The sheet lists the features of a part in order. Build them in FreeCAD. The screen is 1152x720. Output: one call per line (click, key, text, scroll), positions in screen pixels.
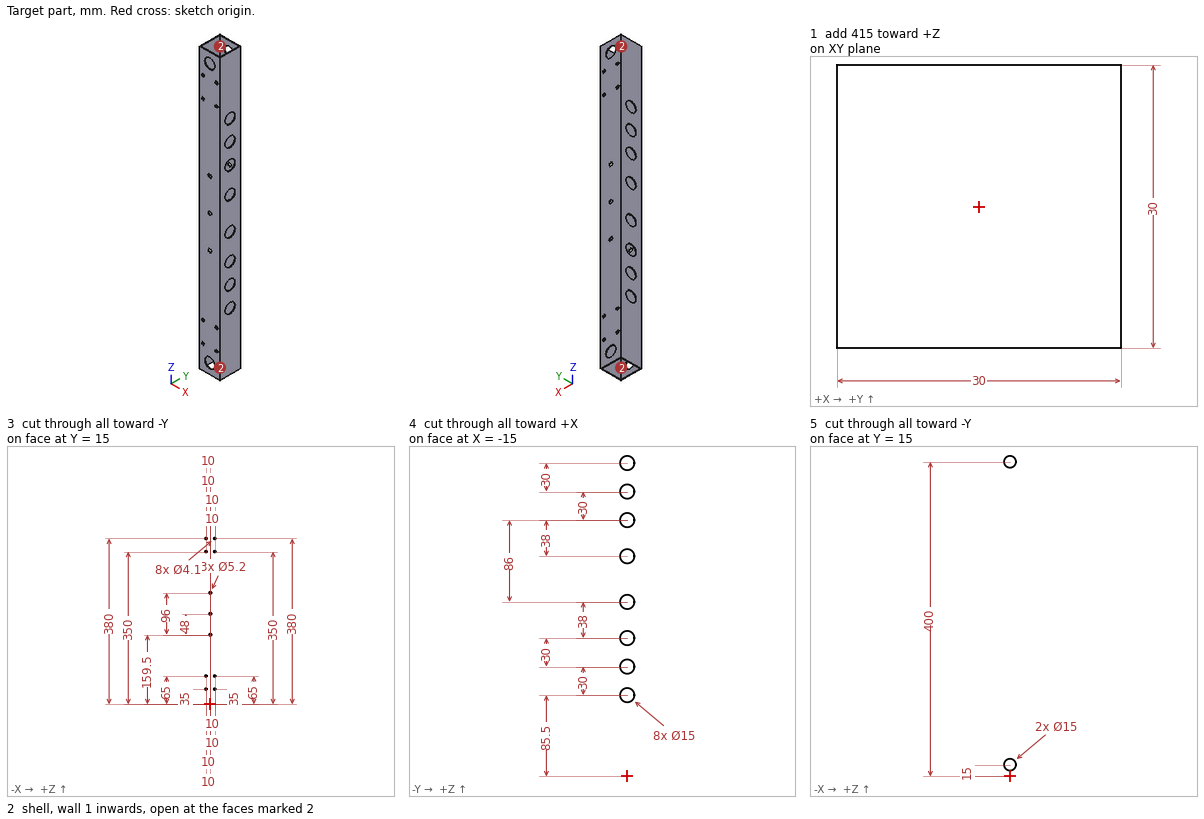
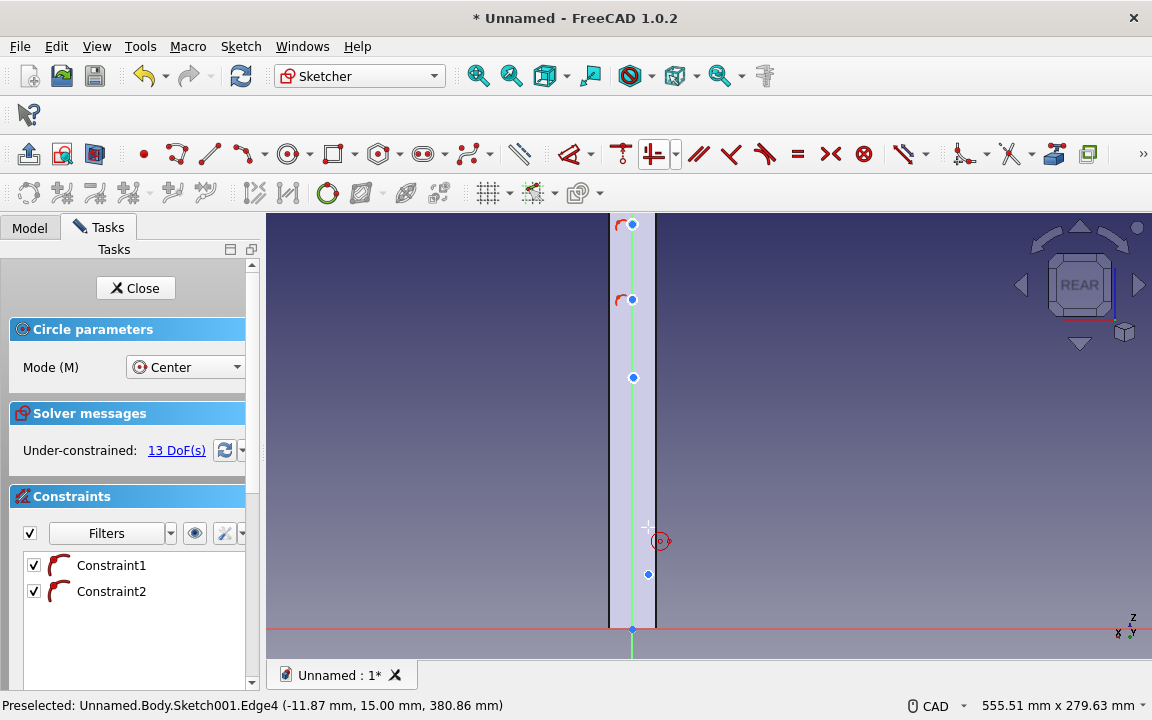
click(648, 526)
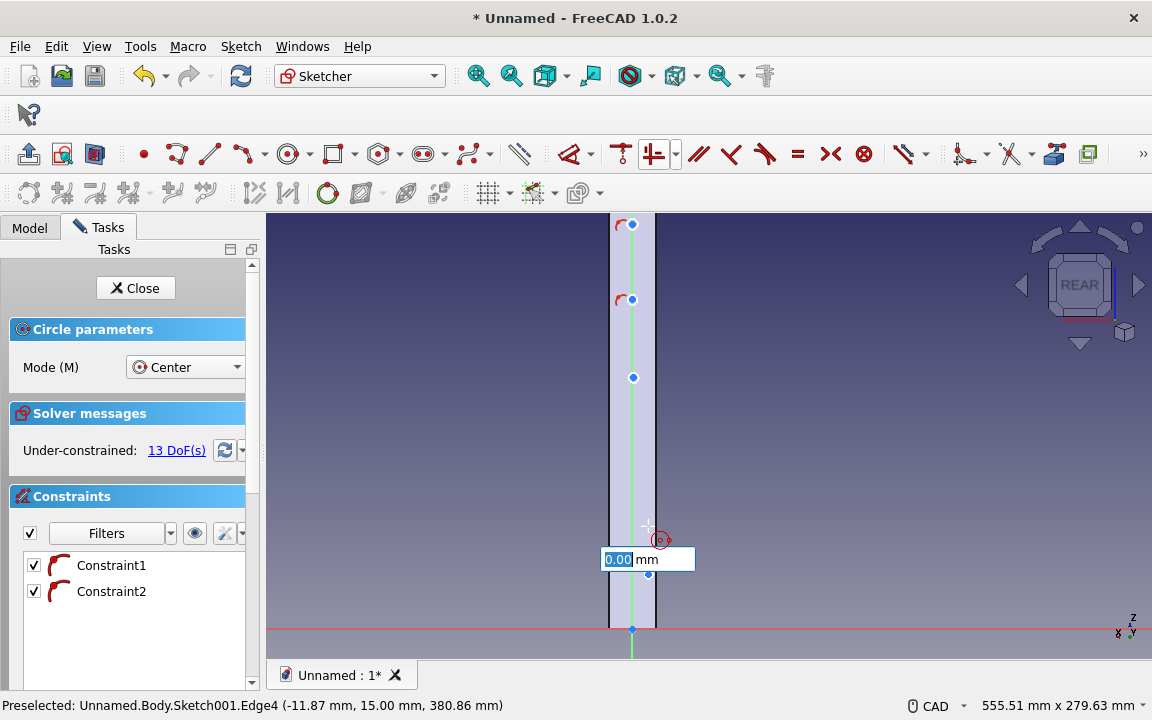
scroll(651, 523, up, 8)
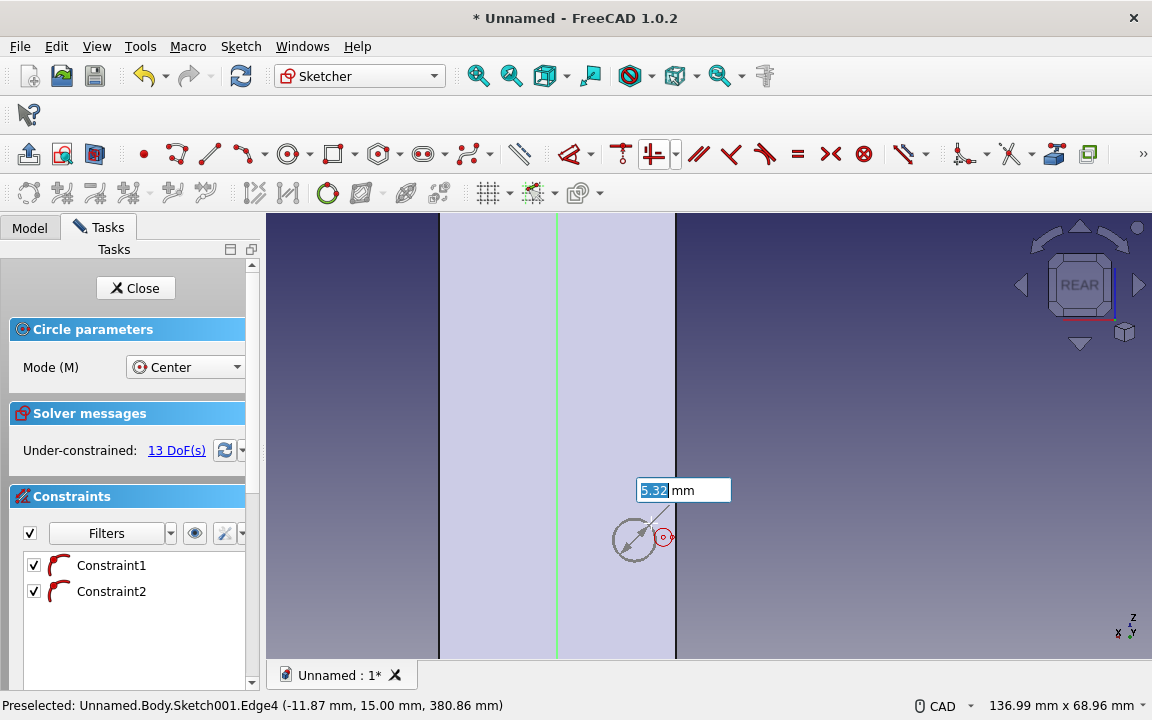
click(648, 522)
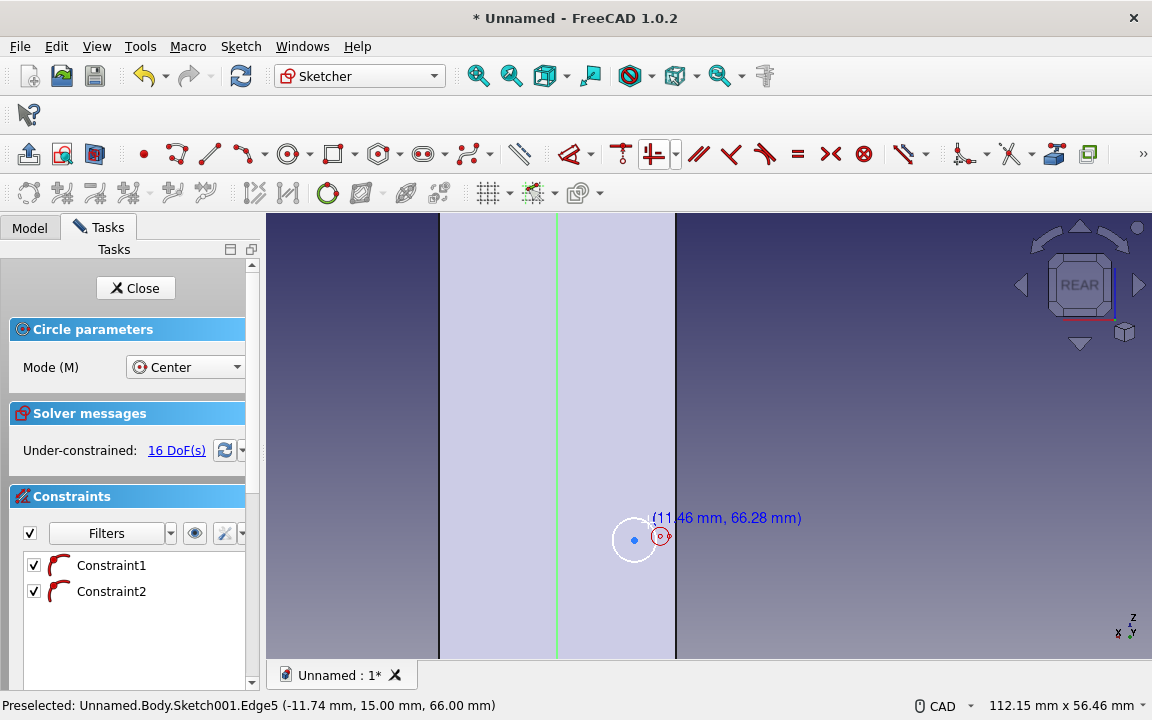
scroll(649, 526, down, 12)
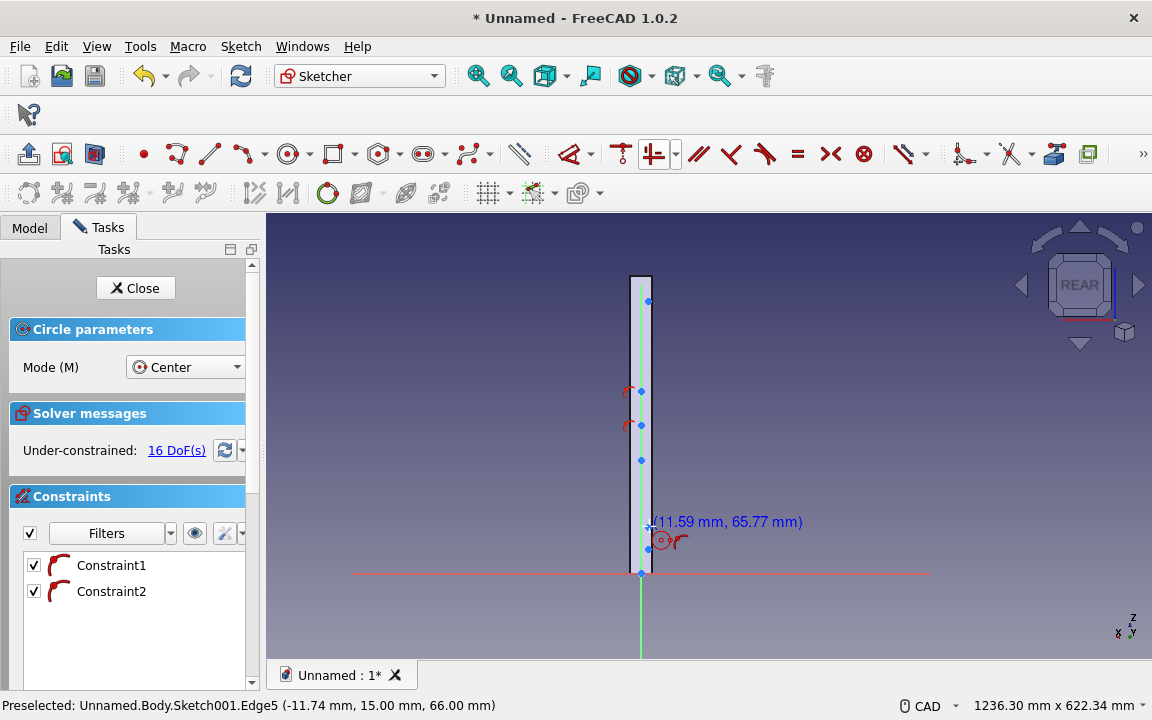
scroll(648, 323, up, 14)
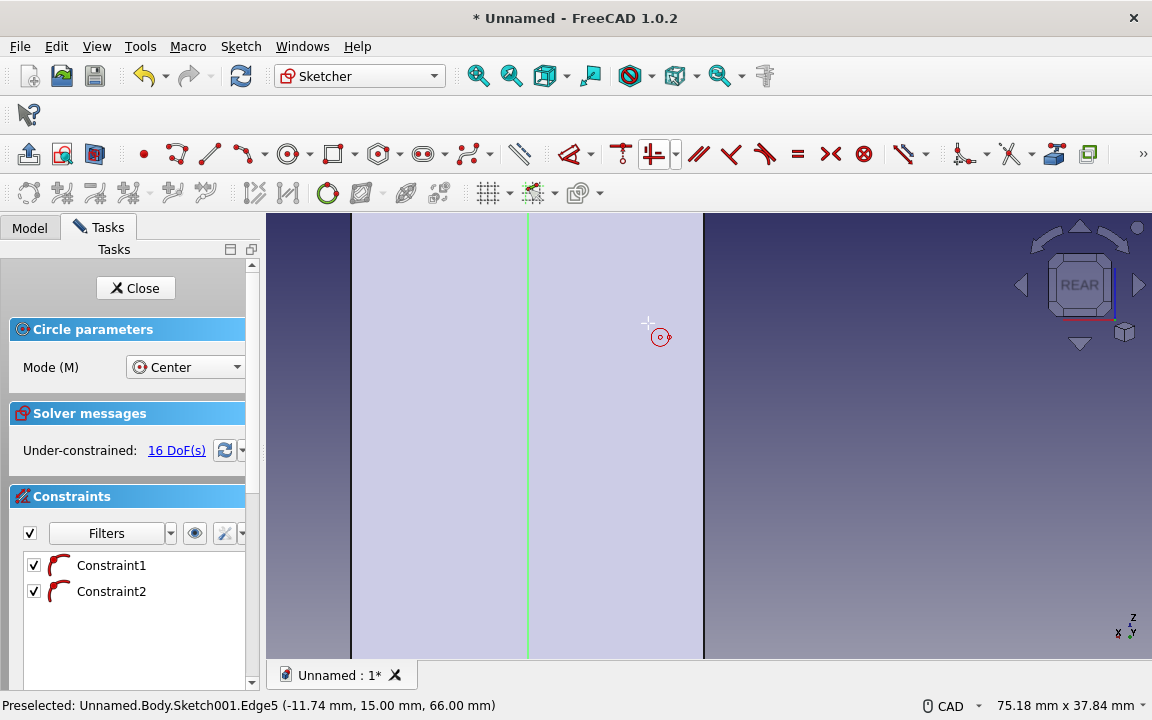
scroll(648, 322, down, 14)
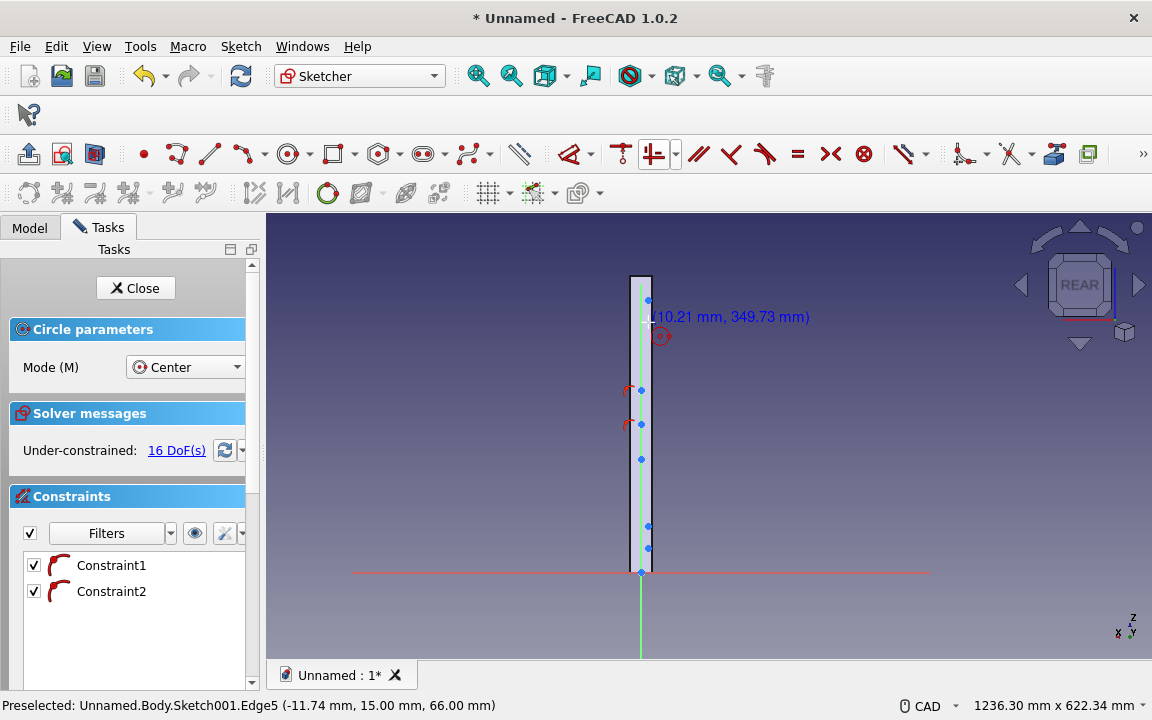
scroll(648, 322, up, 4)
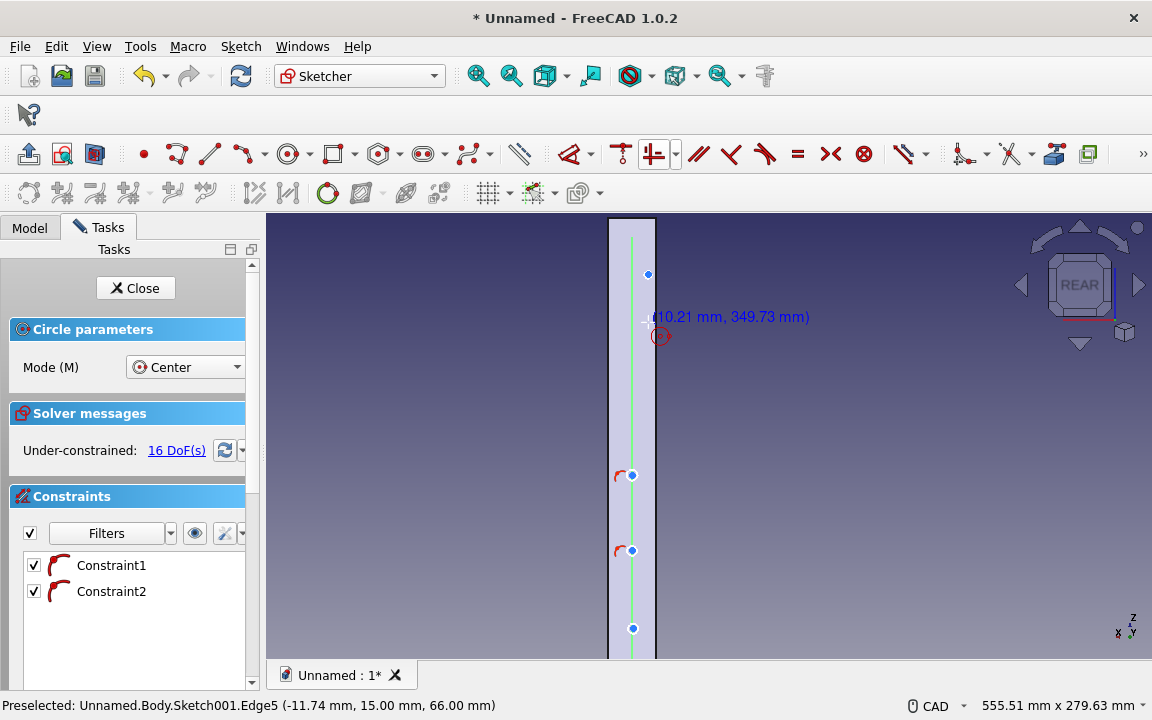
click(648, 322)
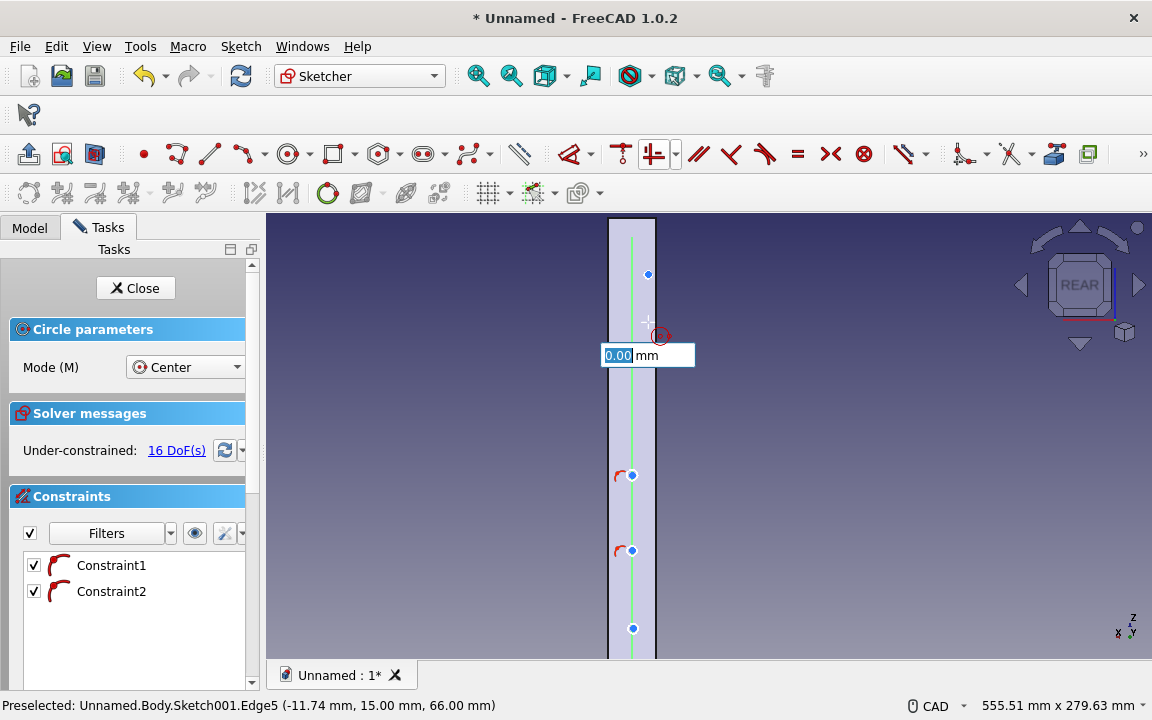
scroll(650, 320, up, 8)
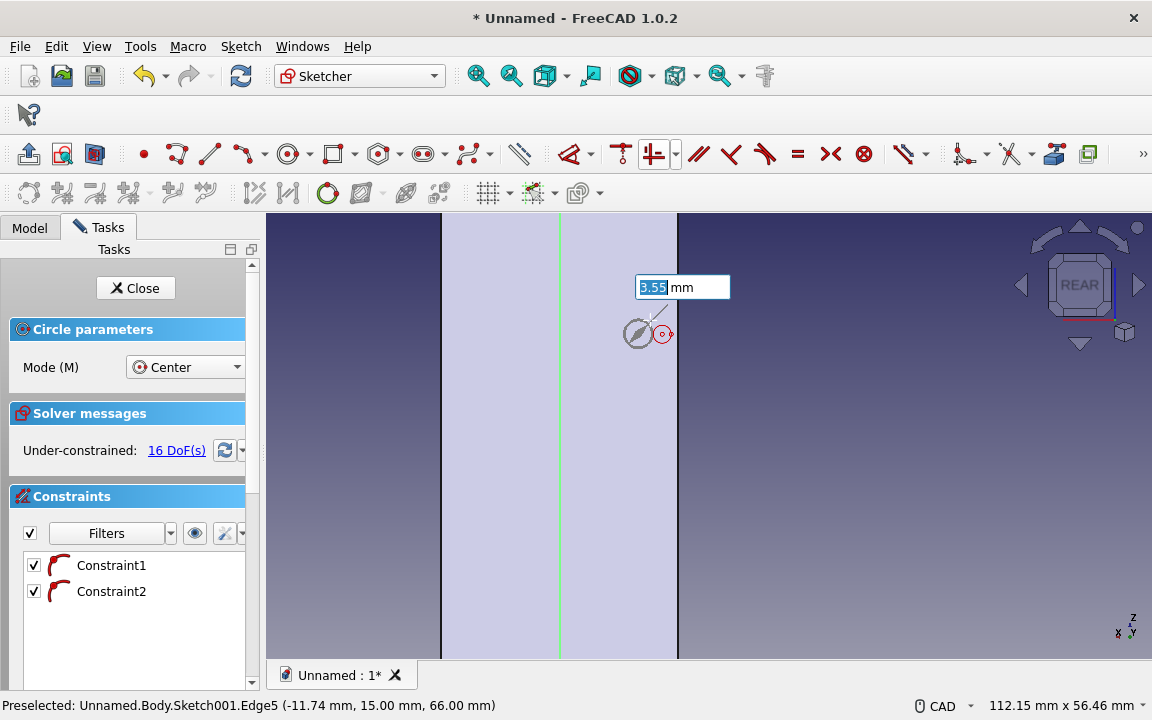
click(650, 317)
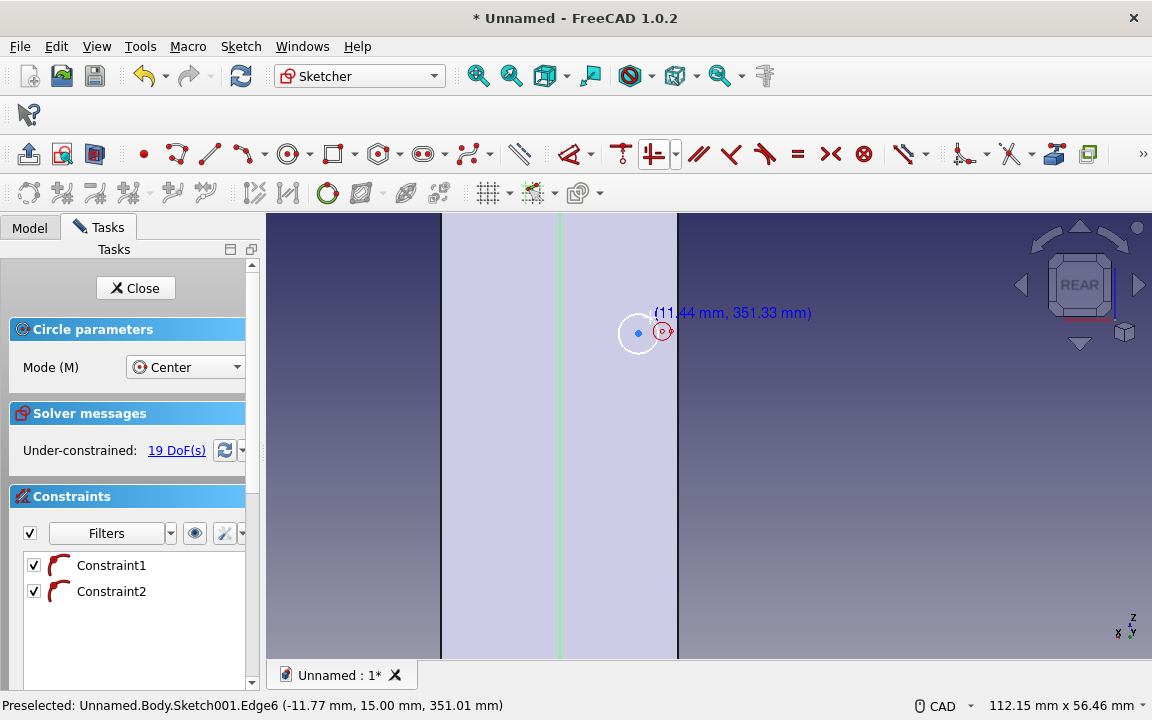
scroll(649, 321, down, 12)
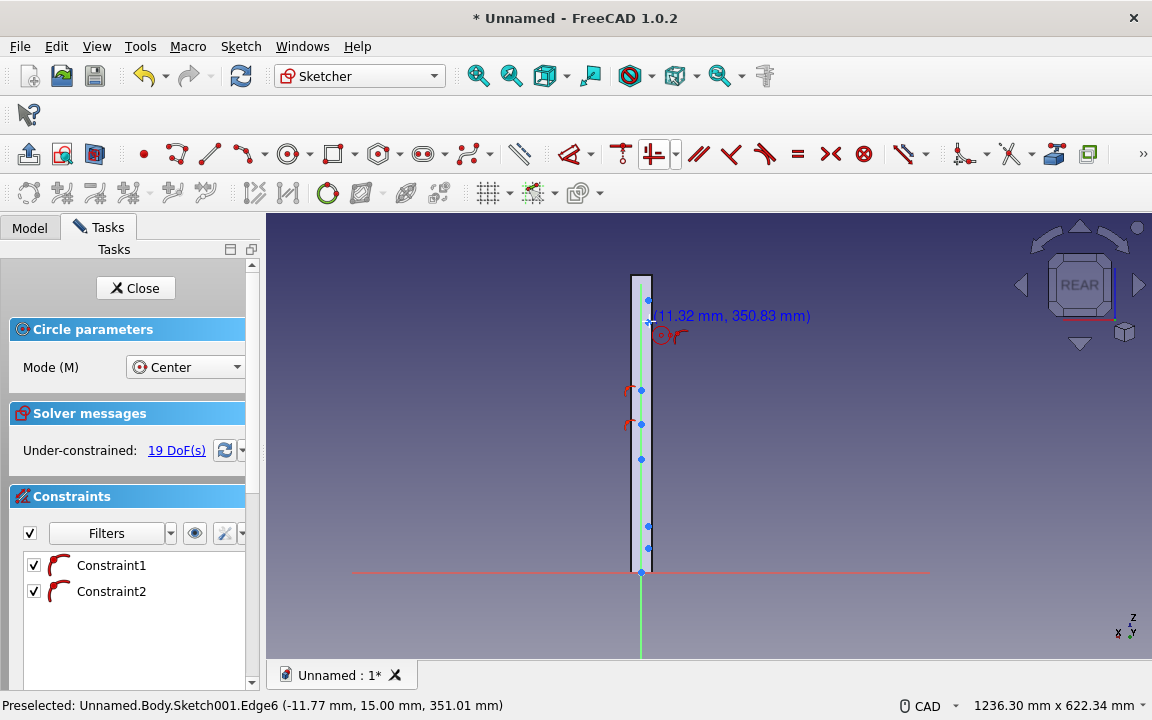
scroll(634, 526, up, 14)